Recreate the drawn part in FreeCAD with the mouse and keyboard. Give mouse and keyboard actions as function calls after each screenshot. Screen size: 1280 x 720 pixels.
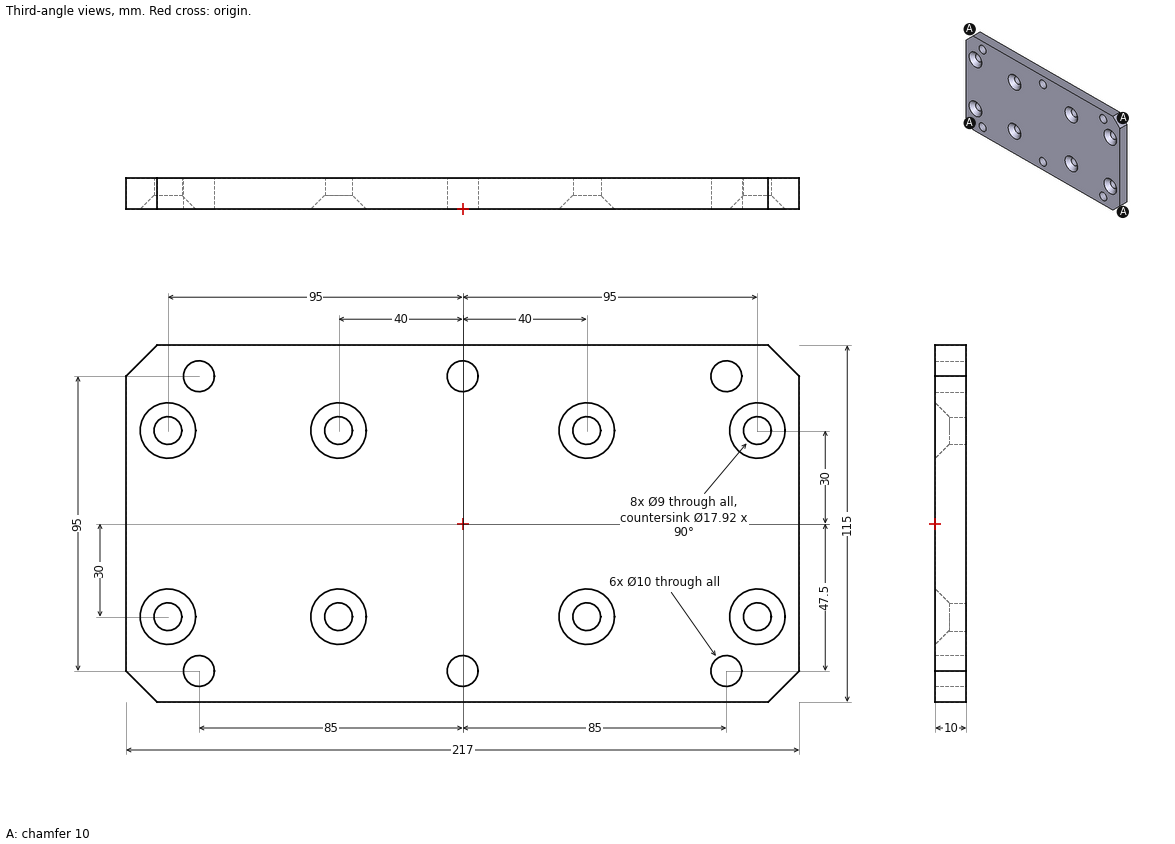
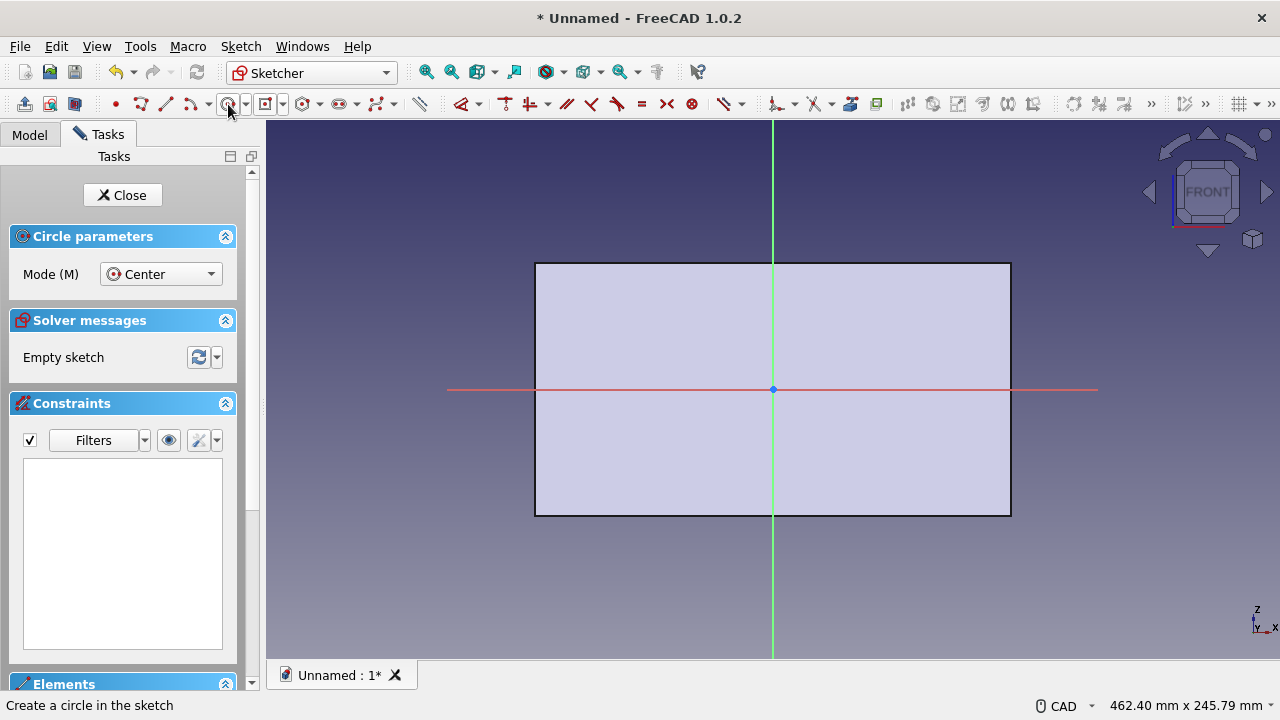
scroll(981, 324, up, 5)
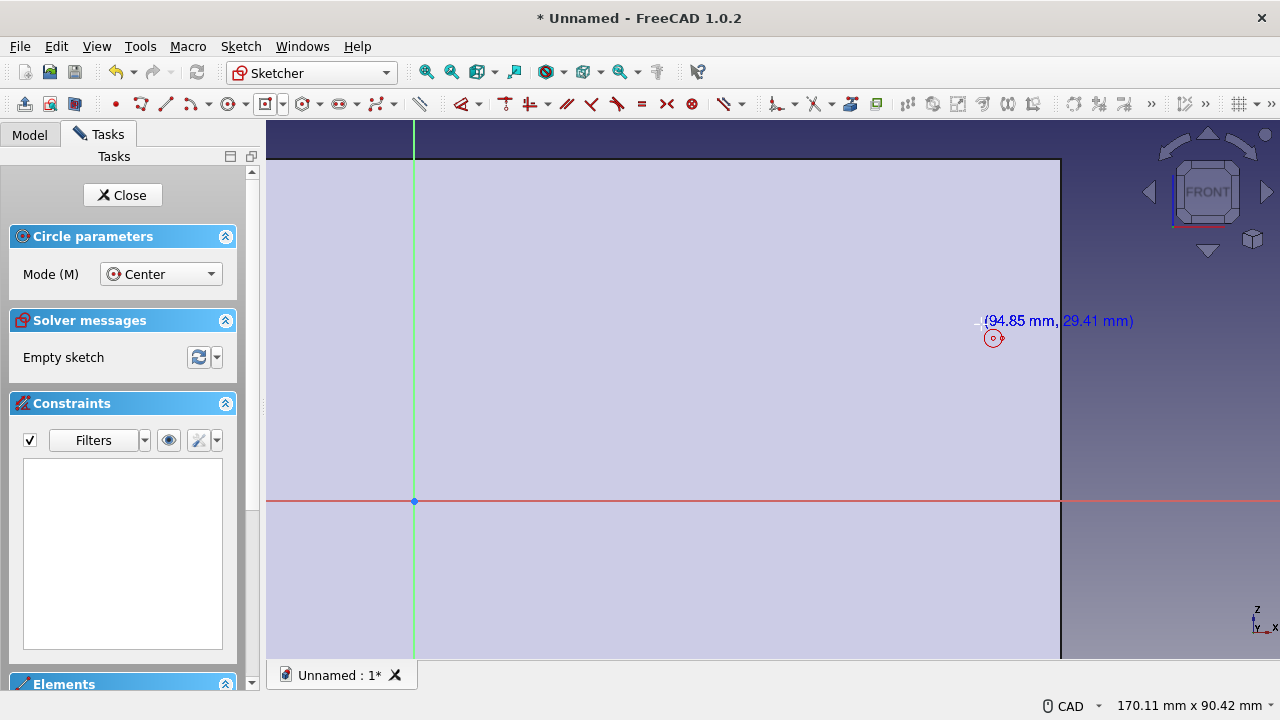
click(981, 323)
click(1000, 304)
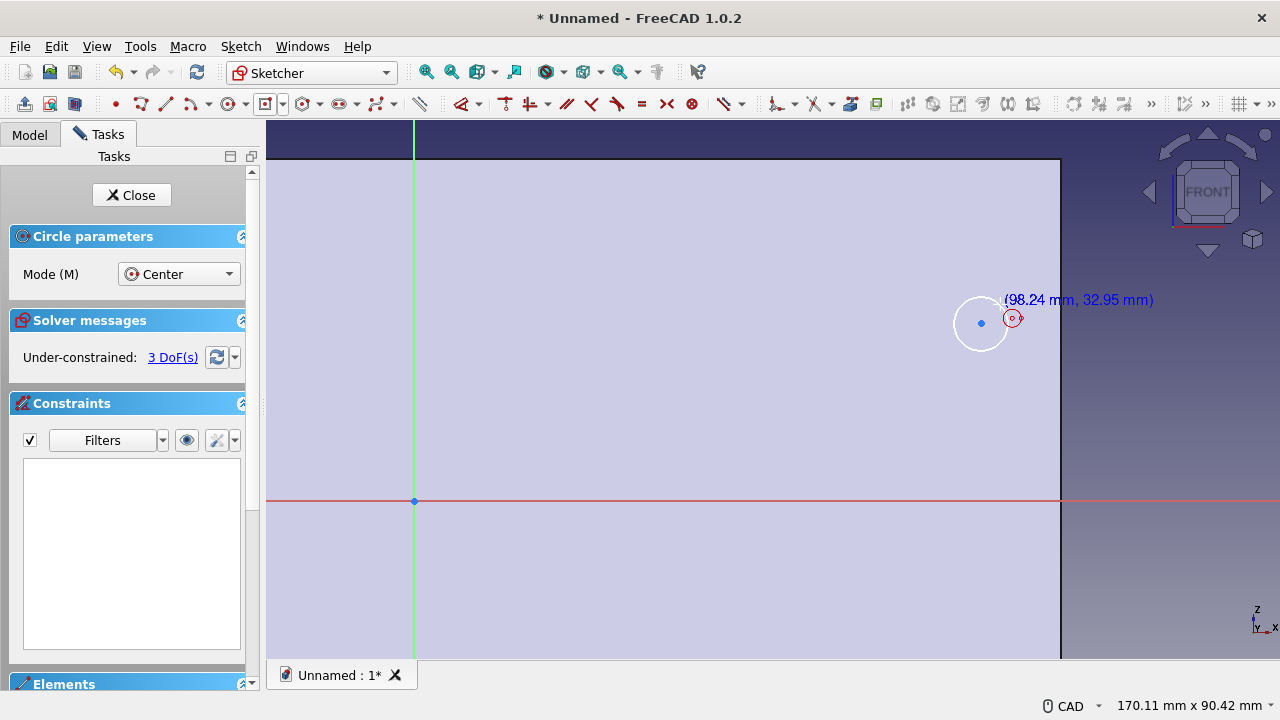
click(653, 323)
click(672, 304)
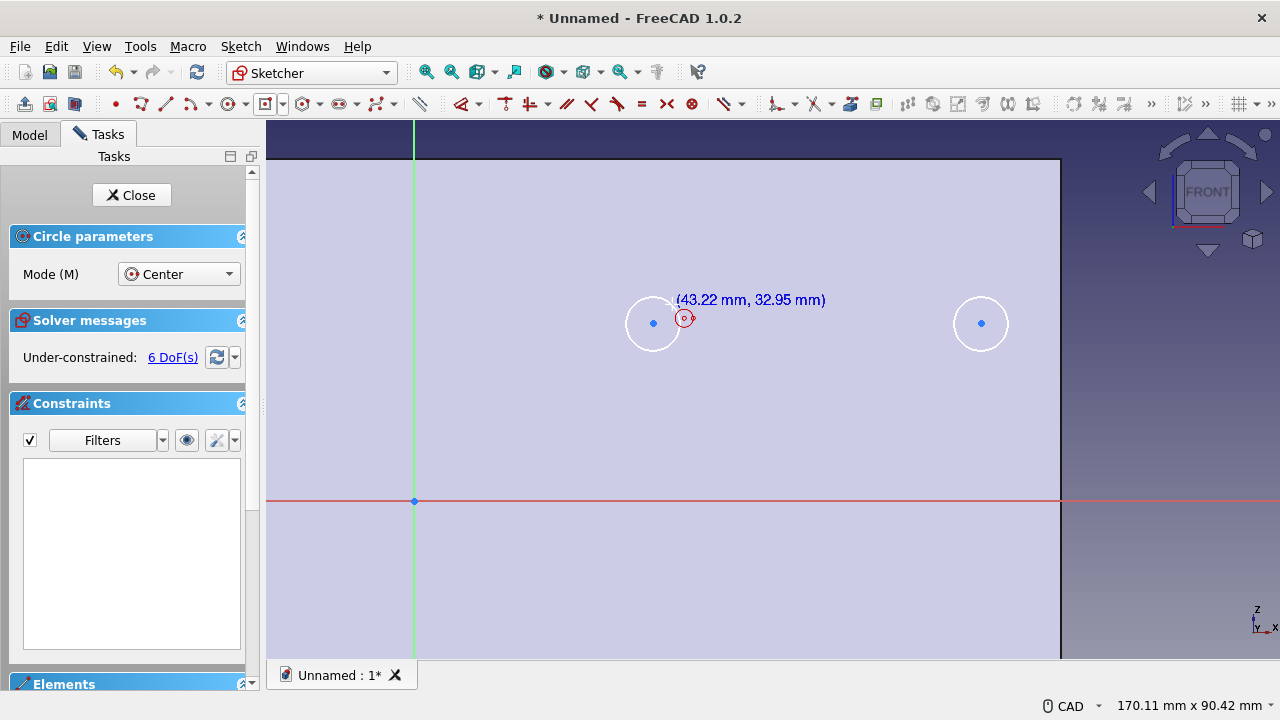
scroll(941, 298, down, 4)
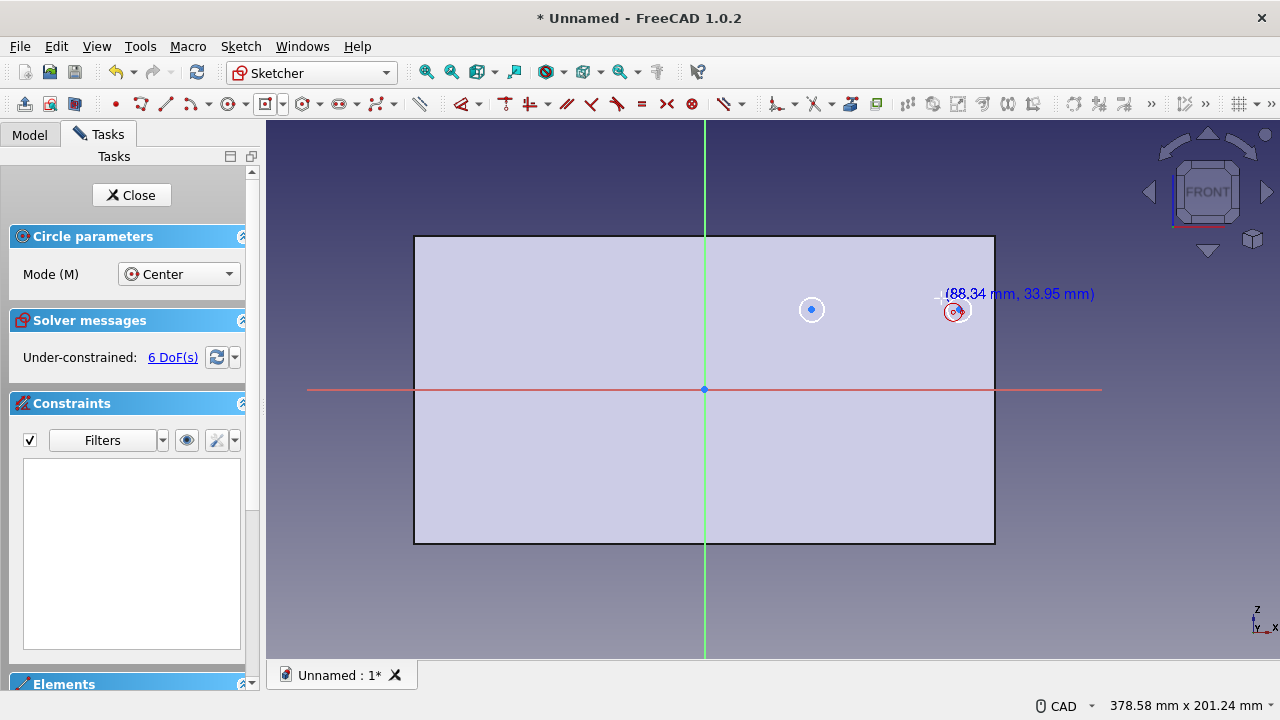
scroll(598, 309, up, 4)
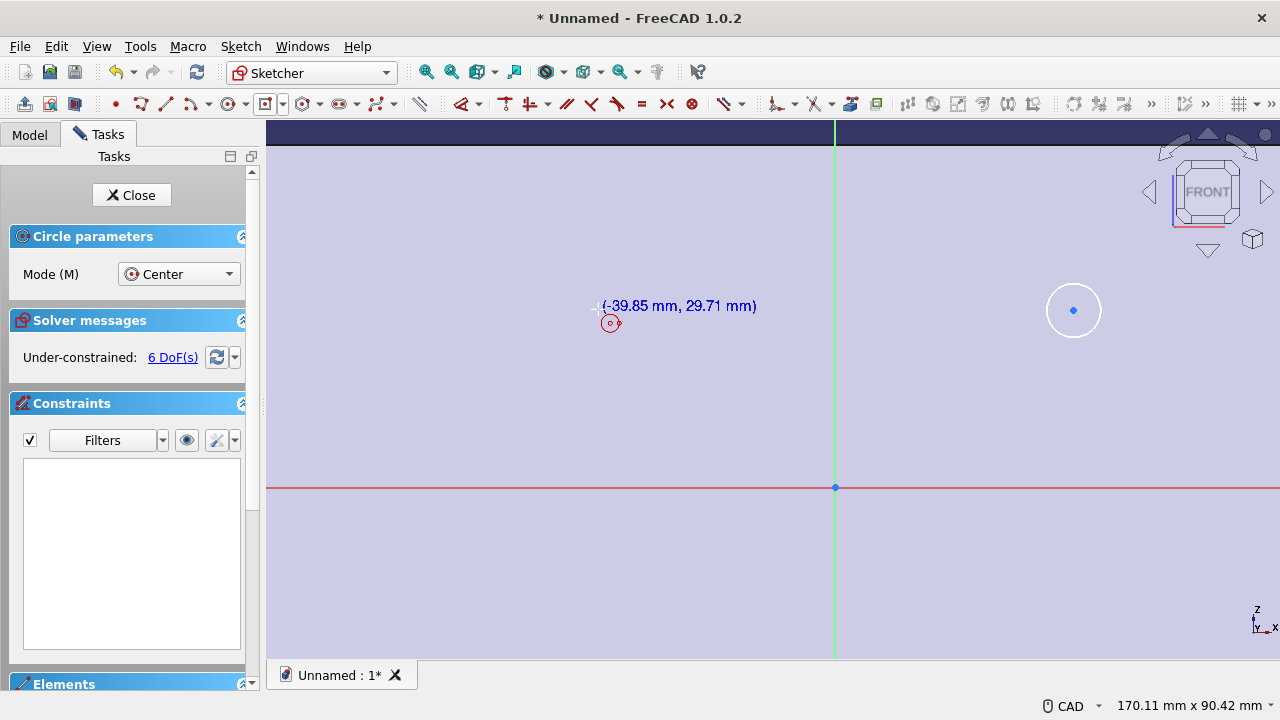
click(597, 309)
click(616, 290)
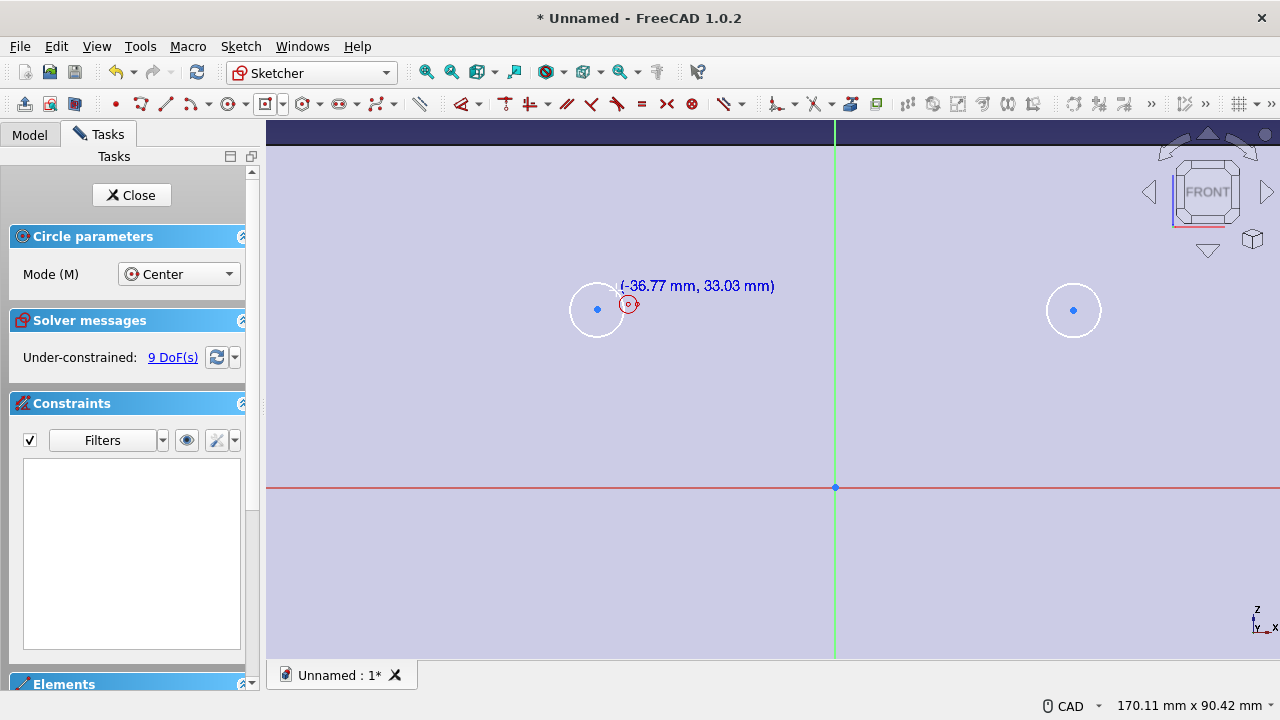
scroll(598, 309, down, 4)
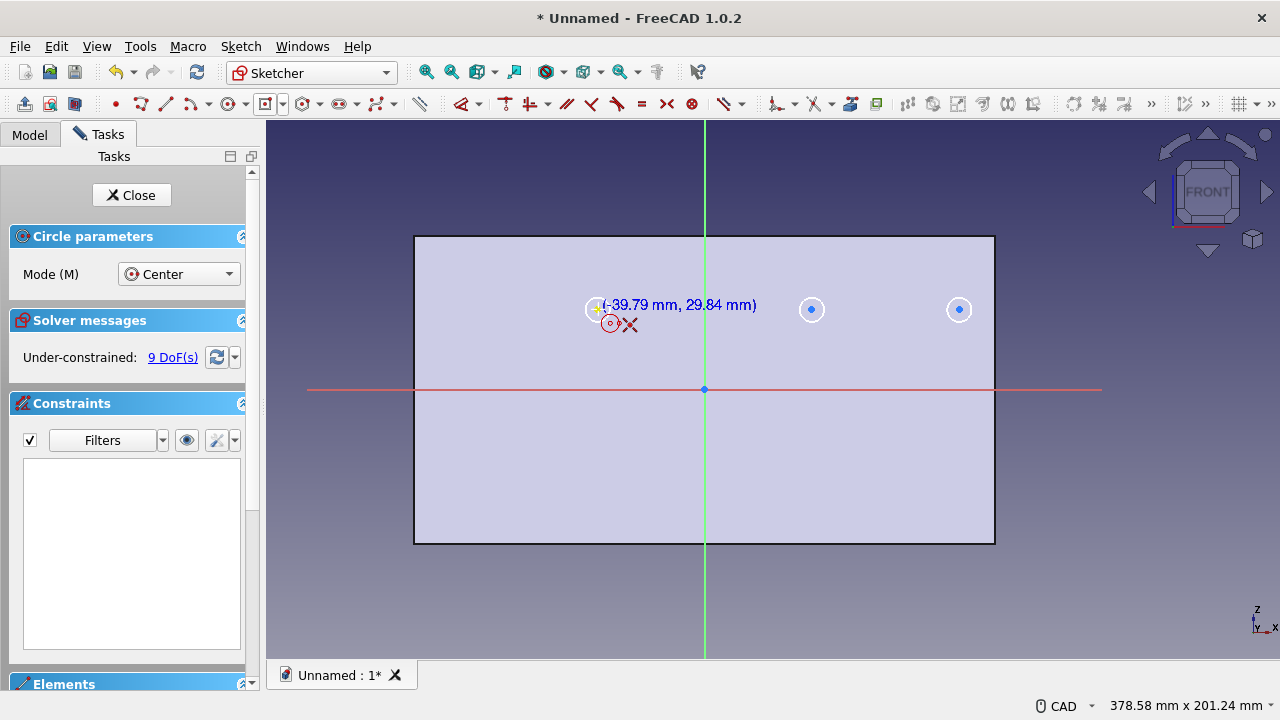
scroll(450, 309, up, 4)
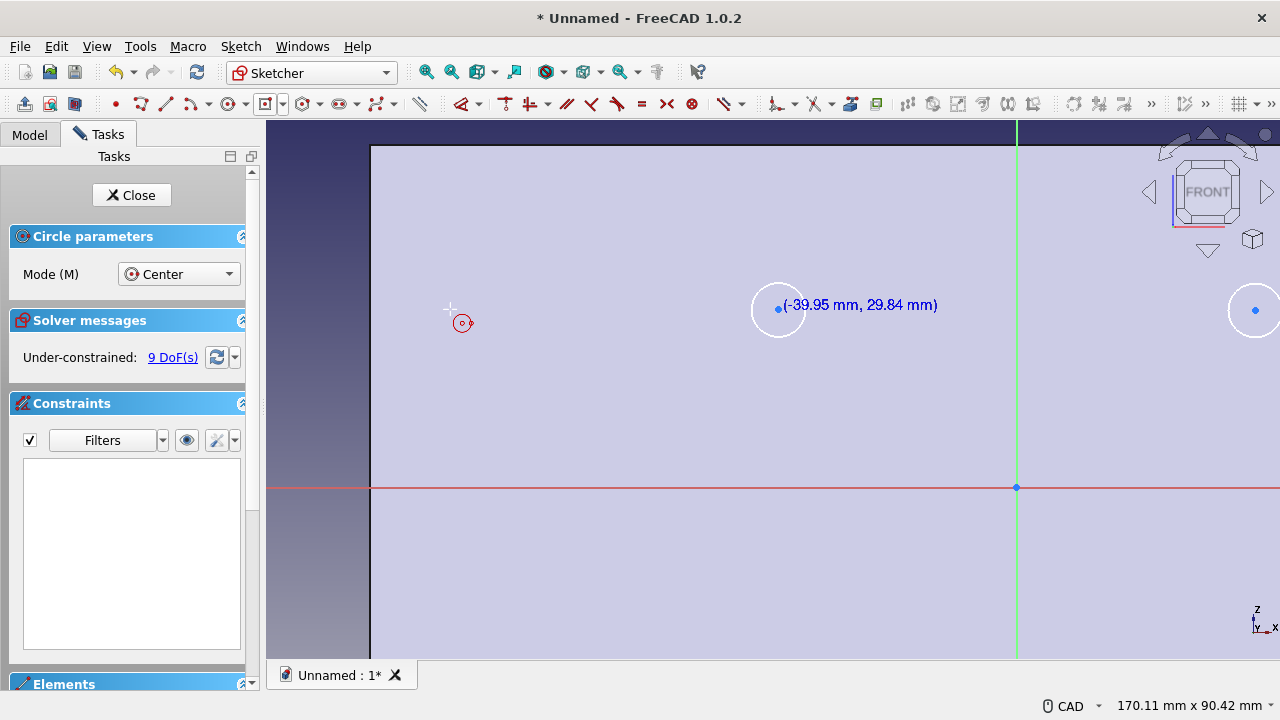
click(450, 309)
click(469, 290)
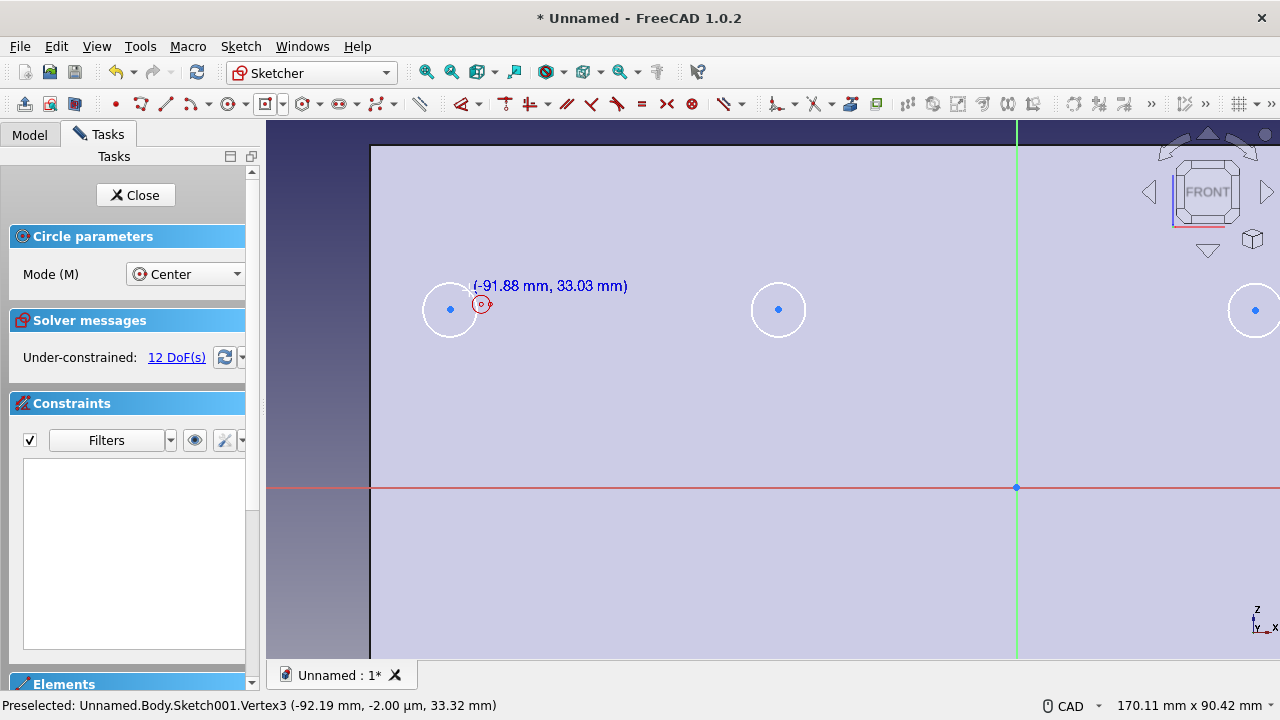
scroll(450, 309, down, 4)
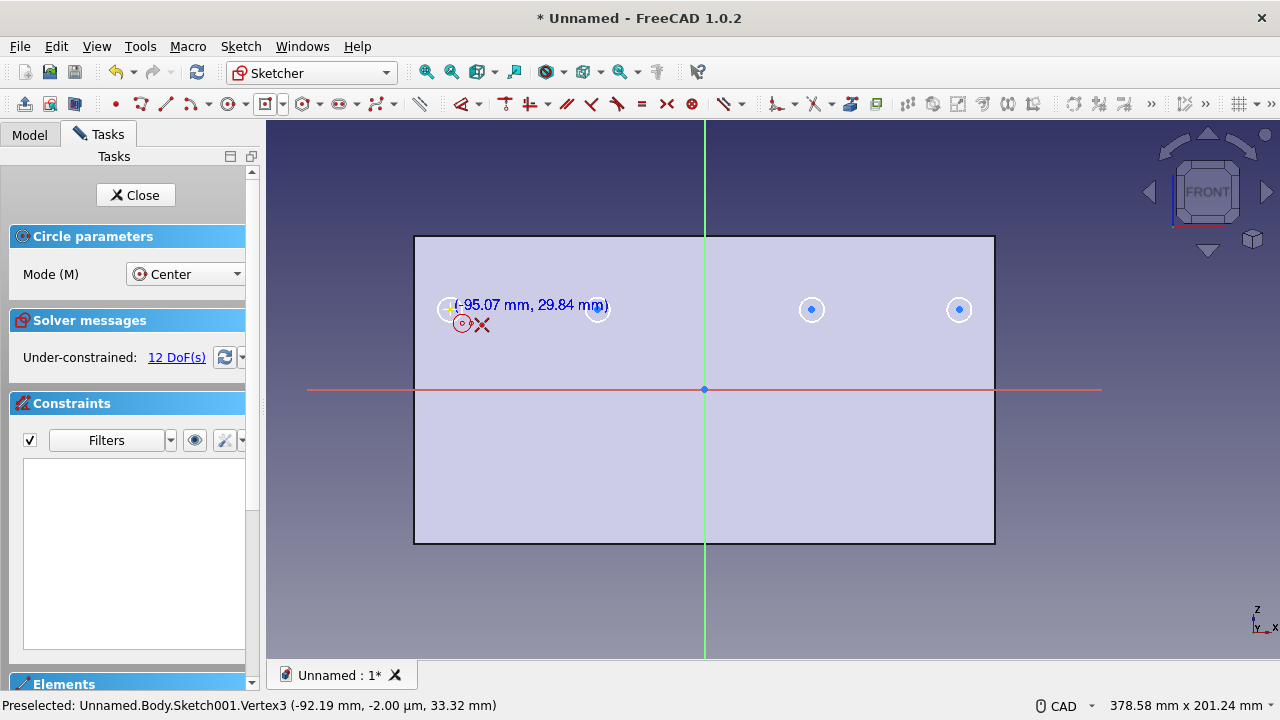
scroll(450, 470, up, 4)